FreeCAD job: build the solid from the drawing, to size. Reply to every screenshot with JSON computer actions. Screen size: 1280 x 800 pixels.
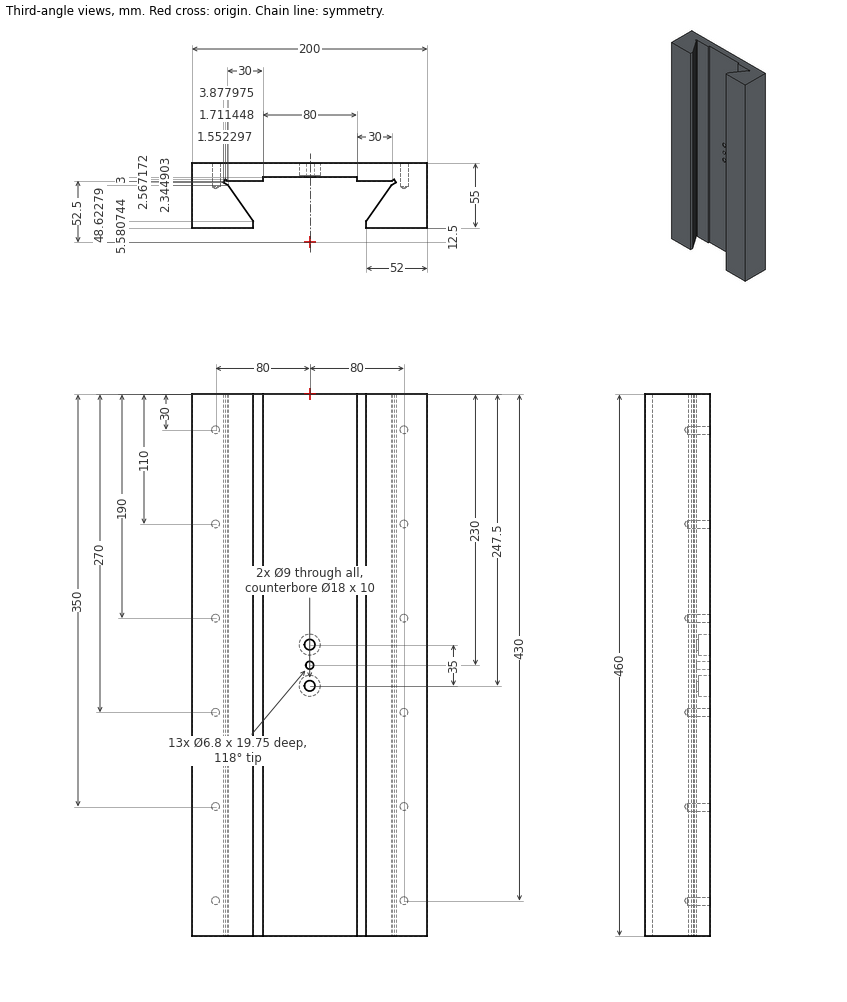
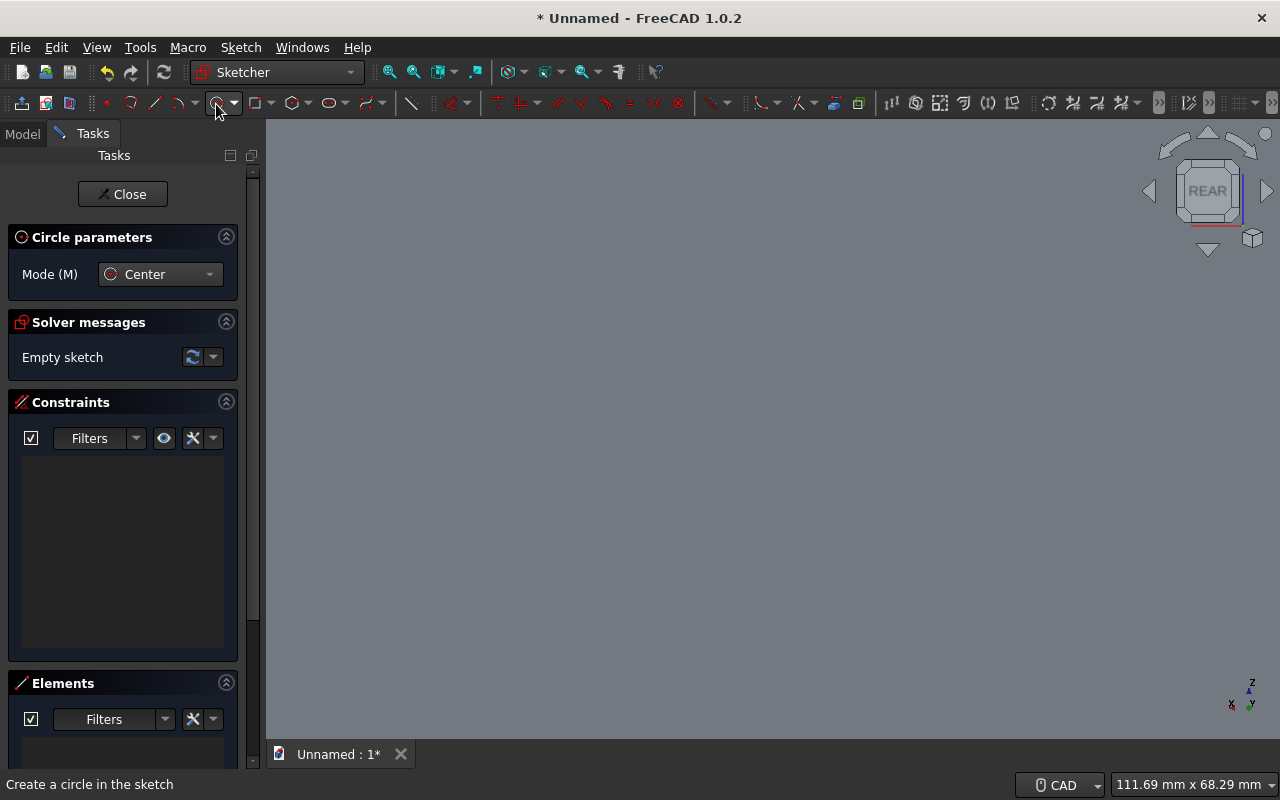
{"action": "left_click", "coordinate": [699, 585]}
{"action": "mouse_move", "coordinate": [728, 556]}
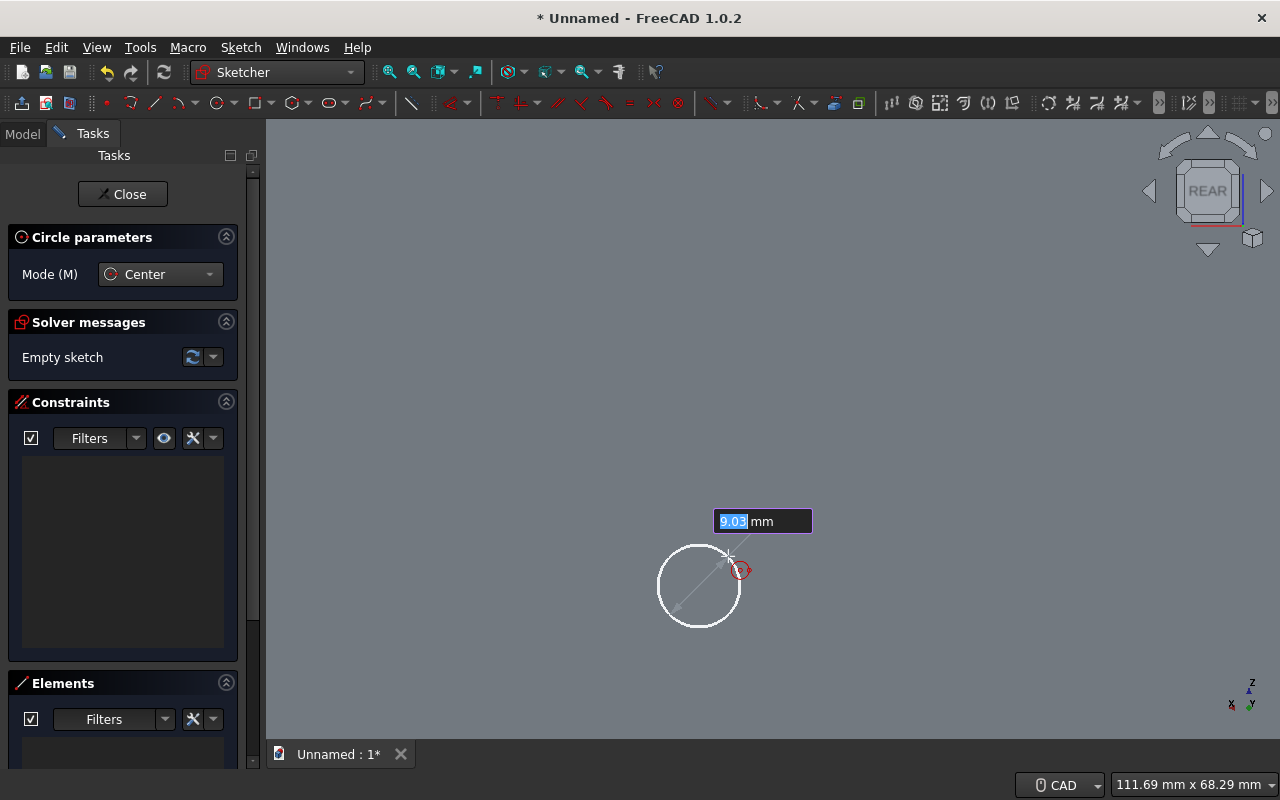
{"action": "type", "text": "9"}
{"action": "key", "text": "Return"}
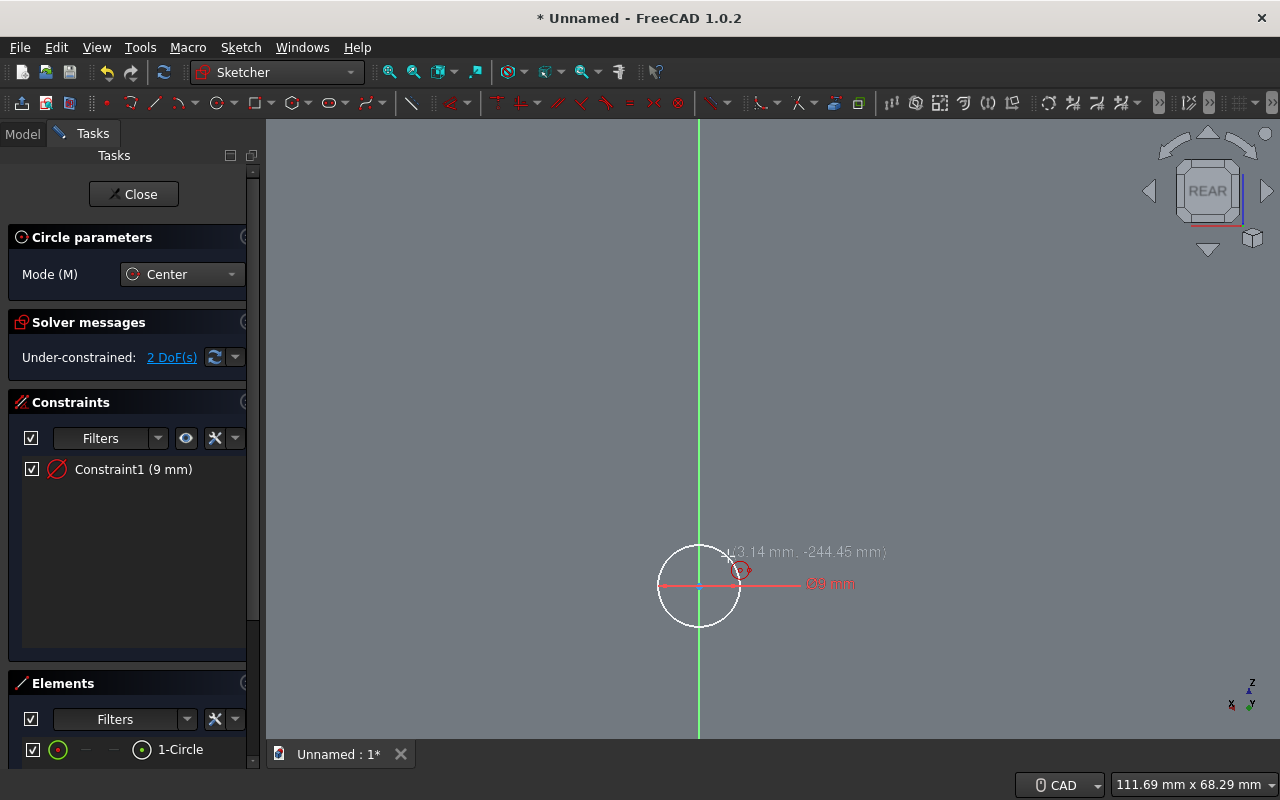
{"action": "left_click", "coordinate": [699, 267]}
{"action": "mouse_move", "coordinate": [728, 238]}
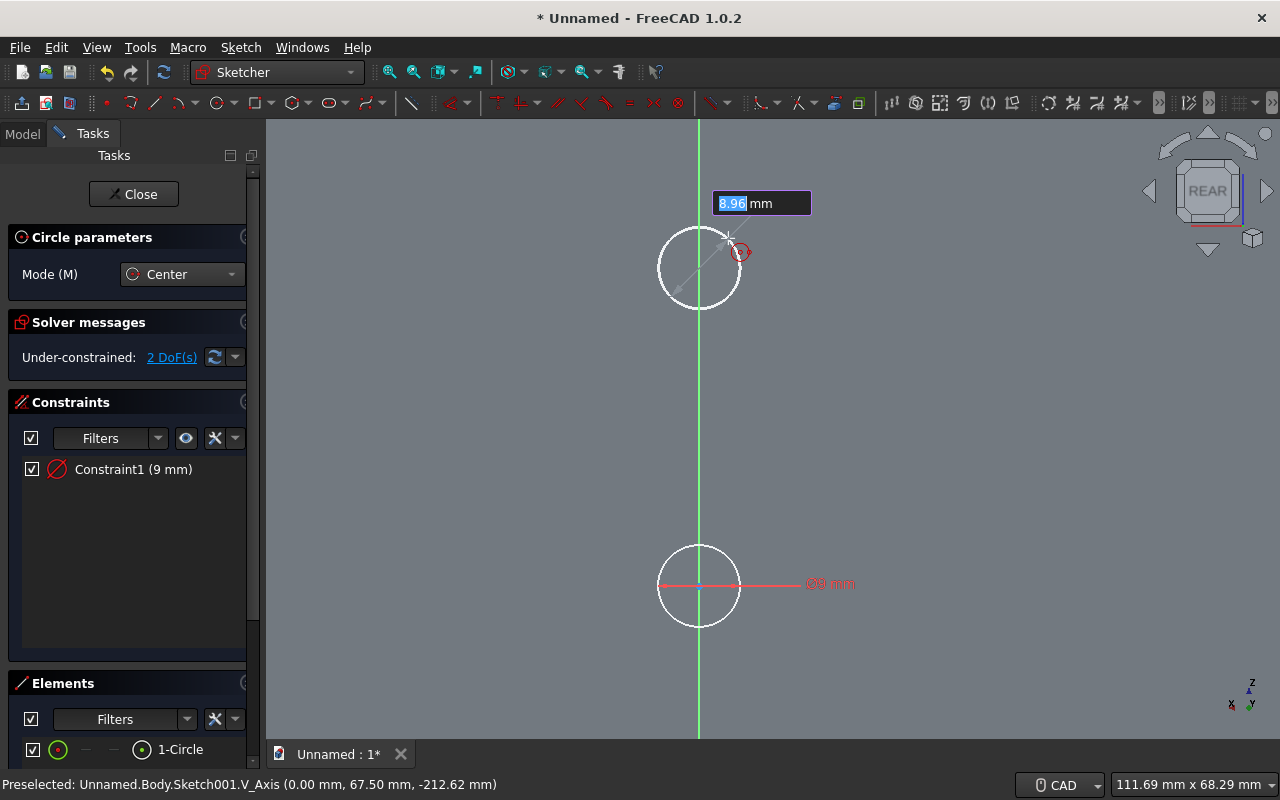
{"action": "type", "text": "9"}
{"action": "key", "text": "Return"}
{"action": "key", "text": "Escape"}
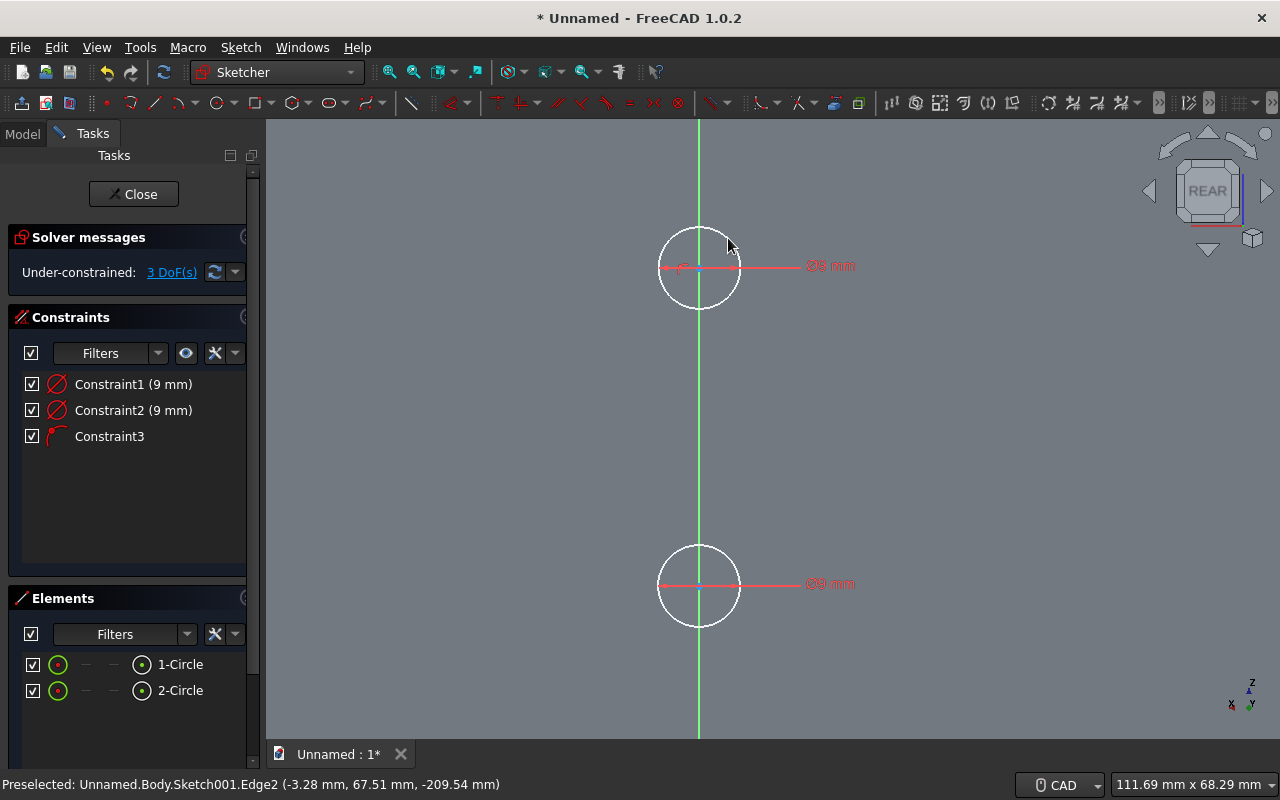
{"action": "left_click", "coordinate": [699, 586]}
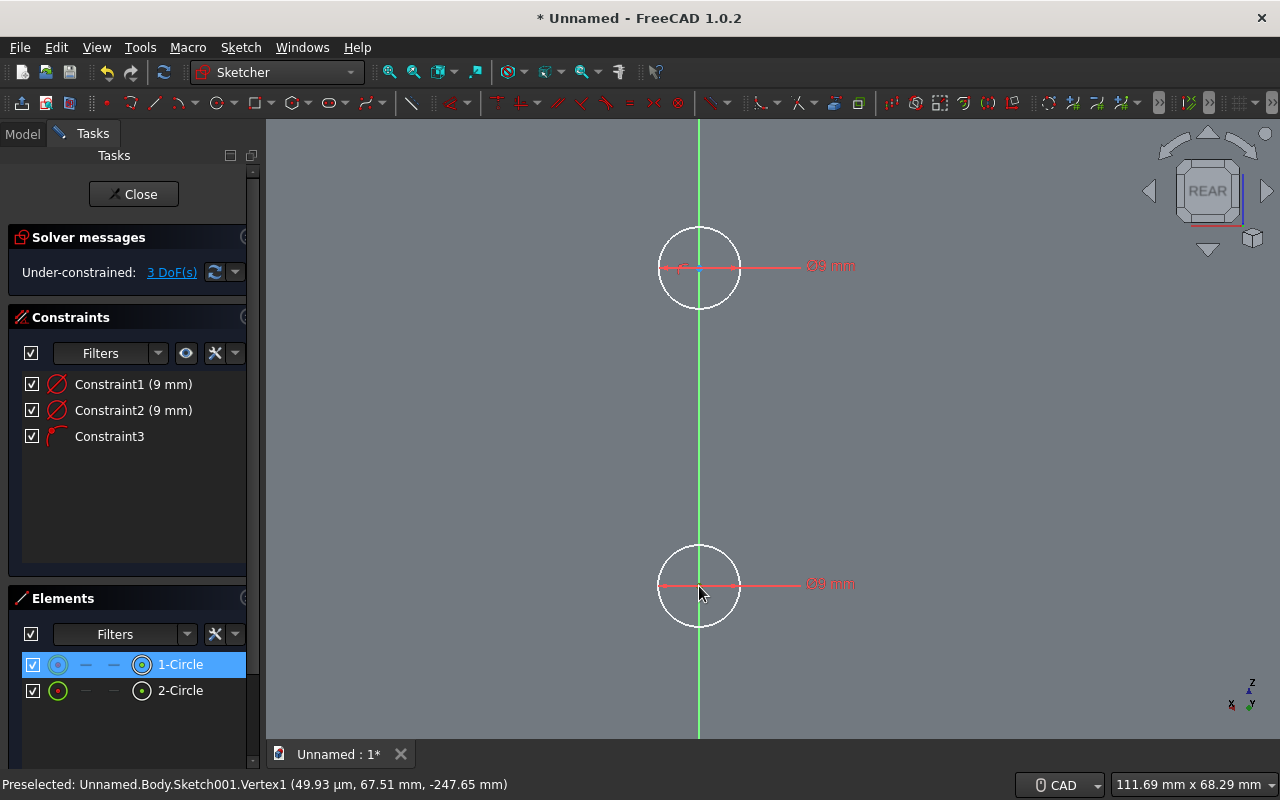
{"action": "left_click", "coordinate": [699, 671]}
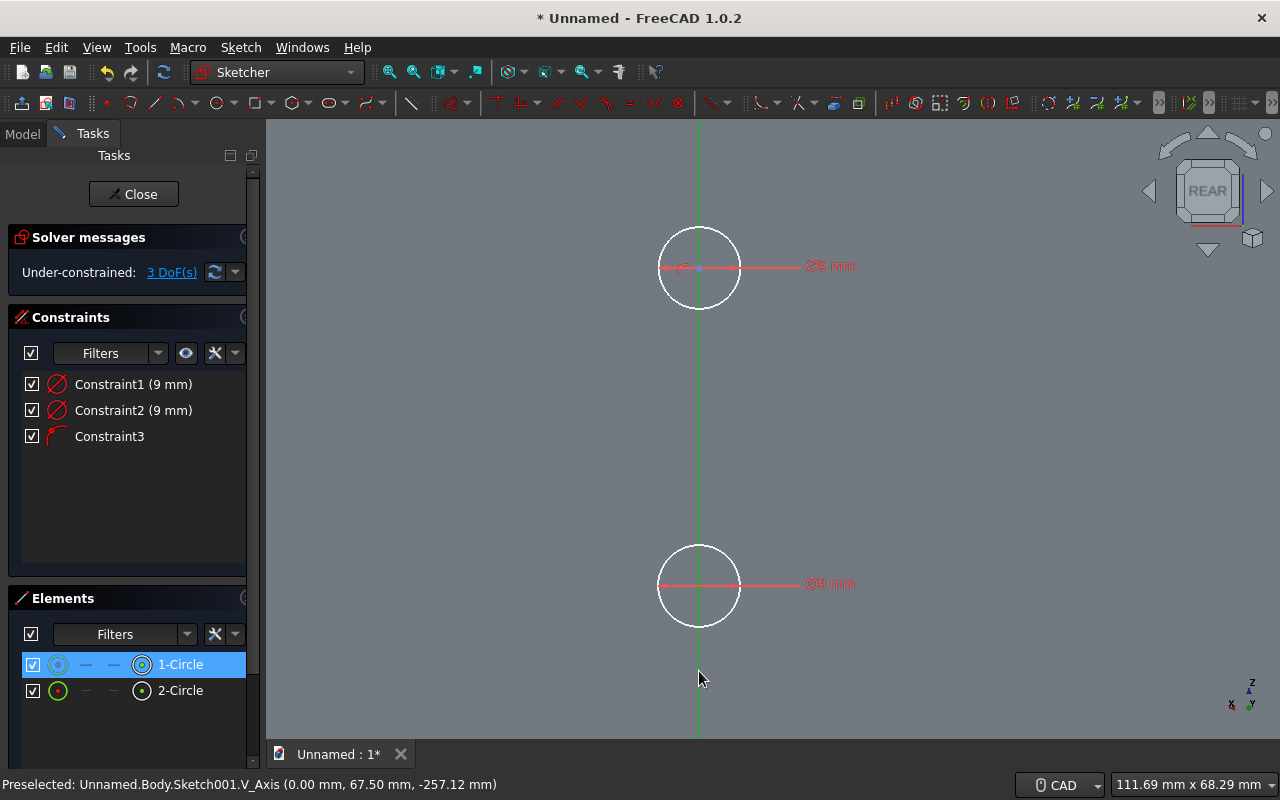
{"action": "left_click", "coordinate": [498, 104]}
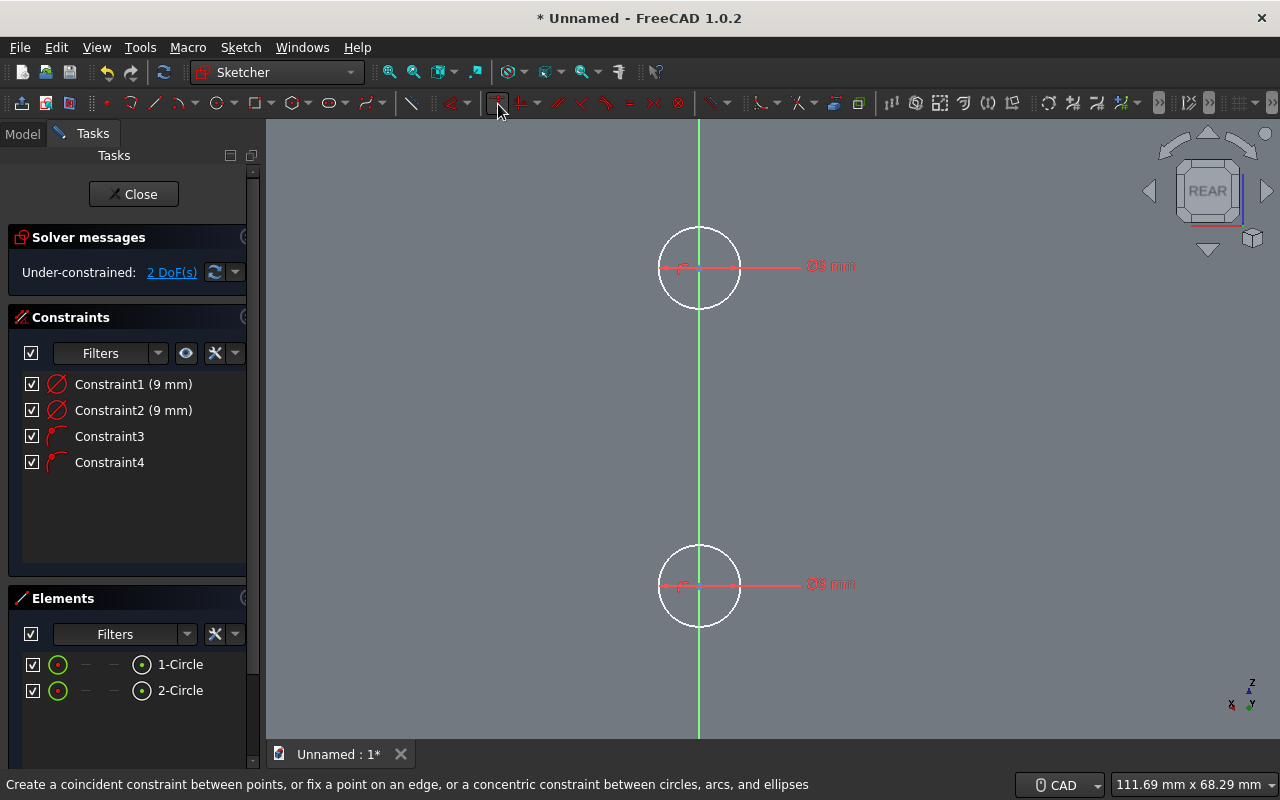
{"action": "left_click", "coordinate": [450, 104]}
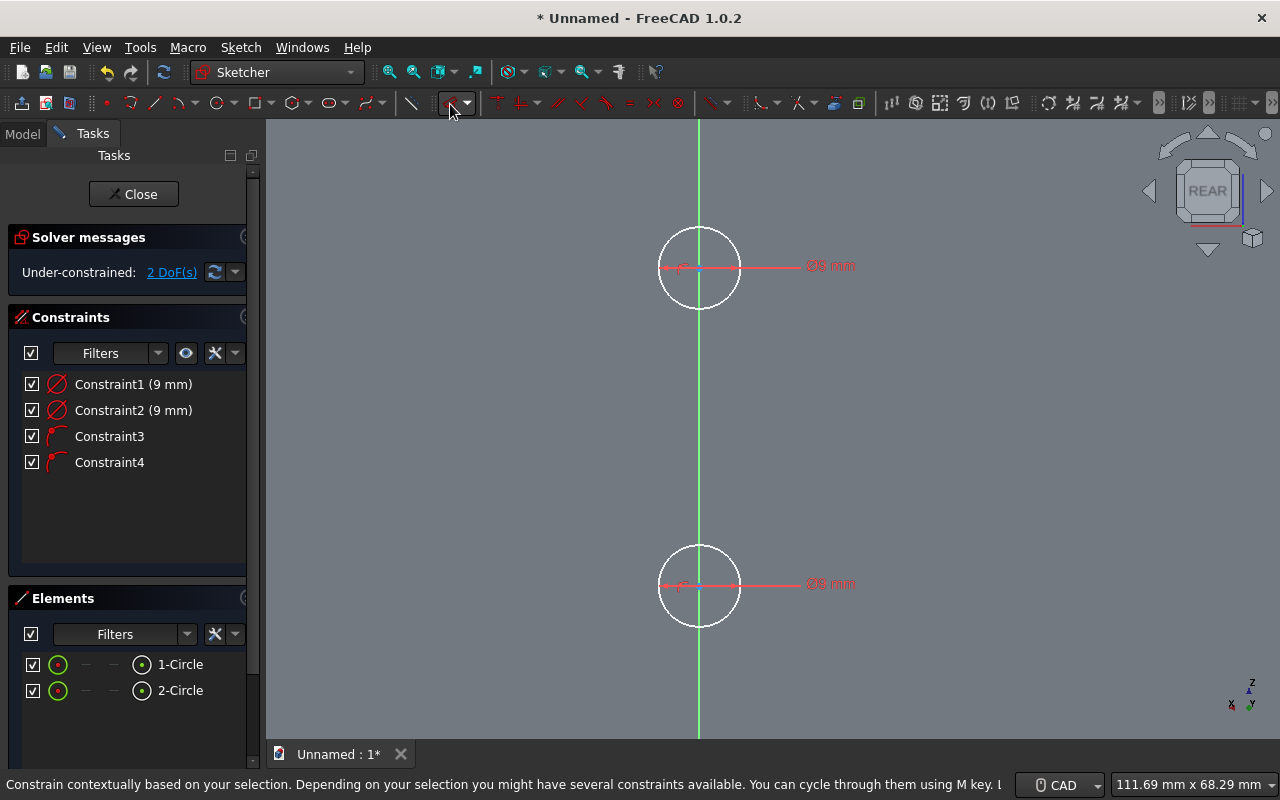
{"action": "left_click", "coordinate": [699, 586]}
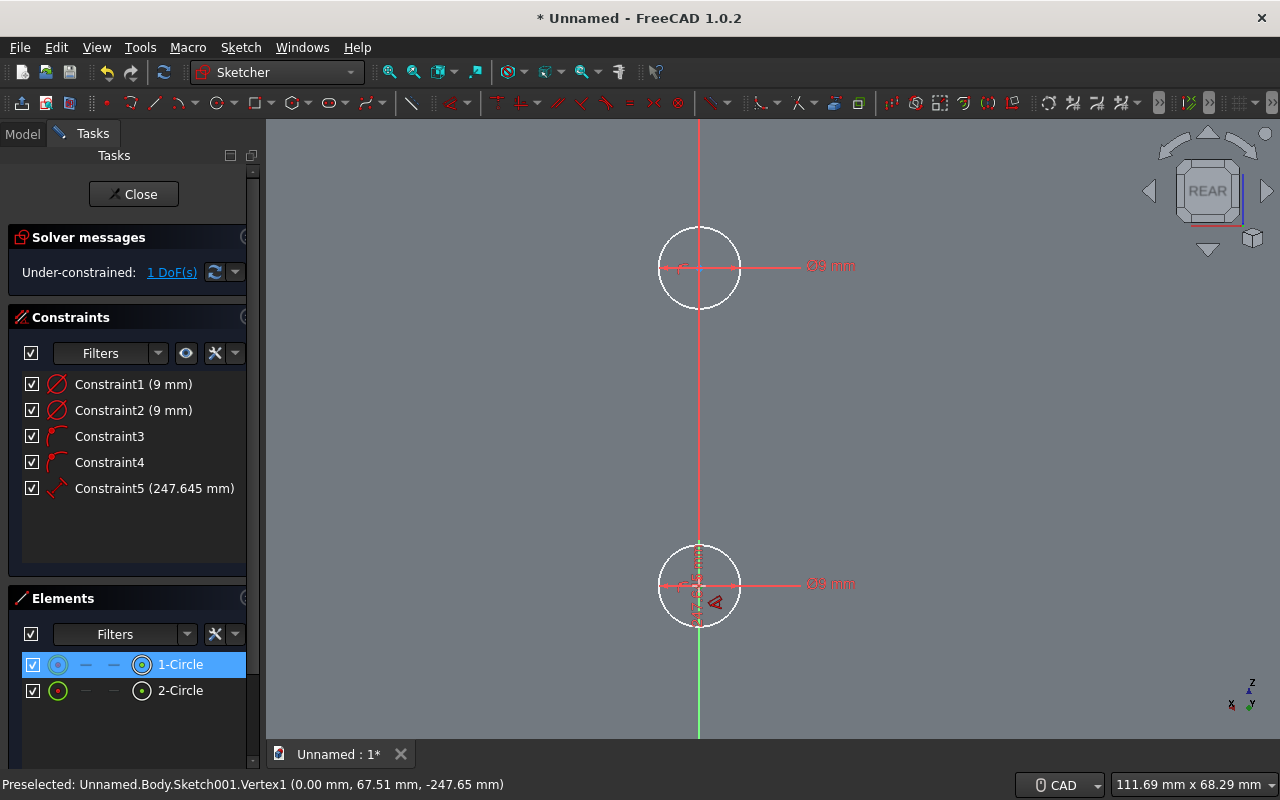
{"action": "left_click", "coordinate": [699, 268]}
{"action": "left_click", "coordinate": [733, 427]}